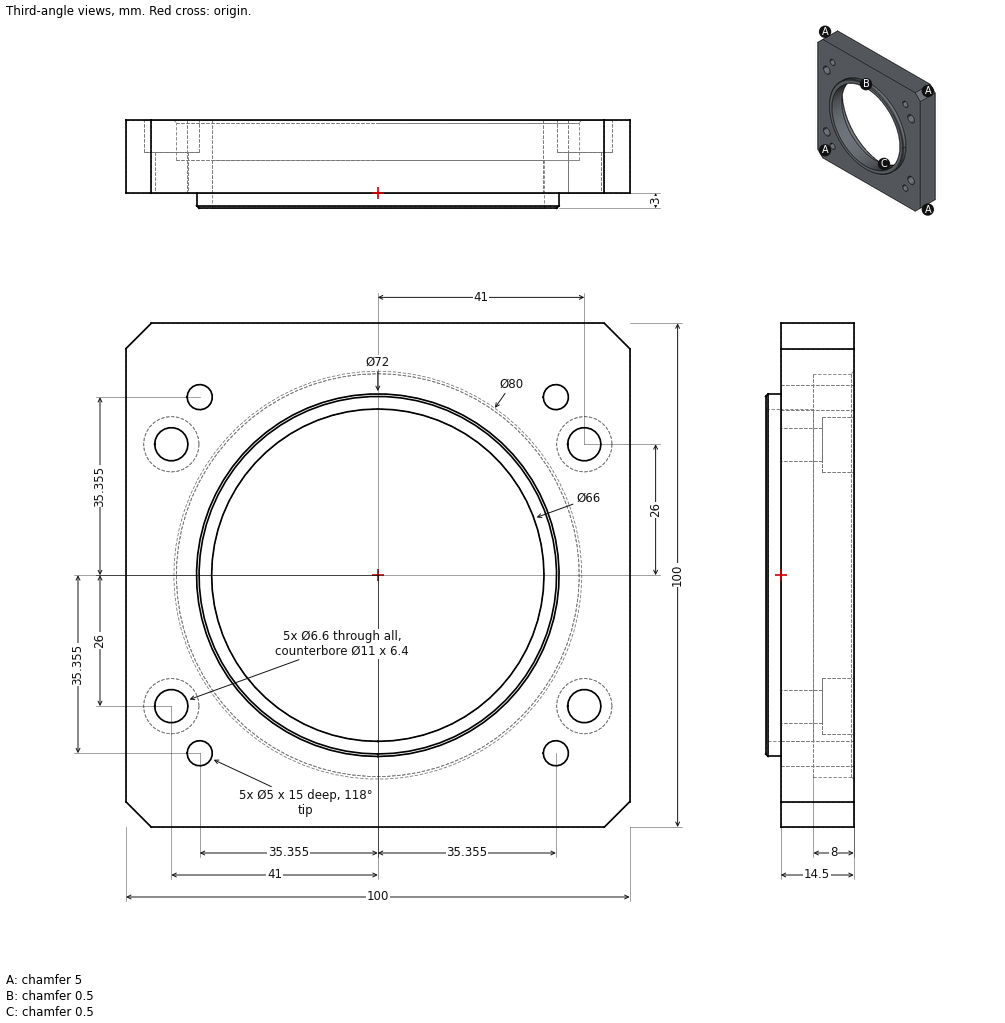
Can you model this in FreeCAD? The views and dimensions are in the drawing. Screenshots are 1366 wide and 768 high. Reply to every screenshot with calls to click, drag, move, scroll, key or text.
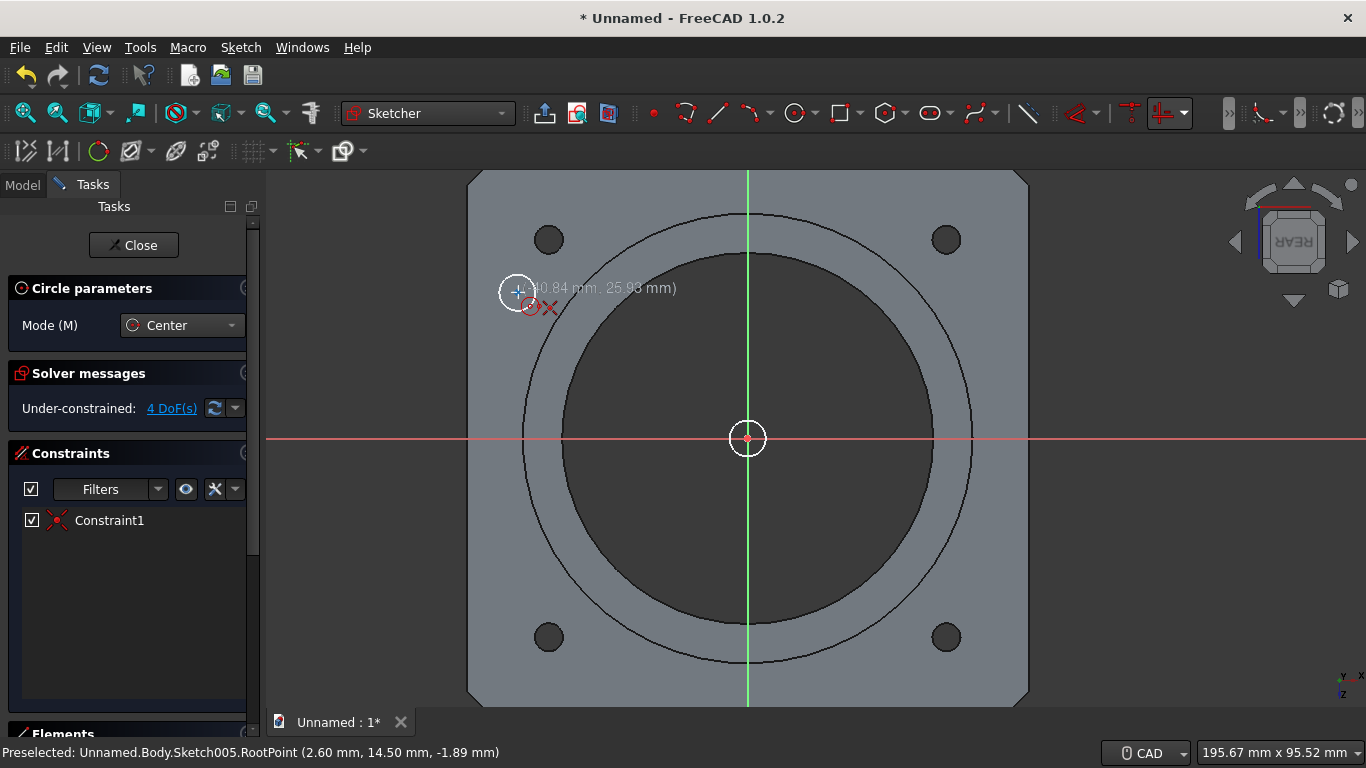
scroll(978, 585, up, 2)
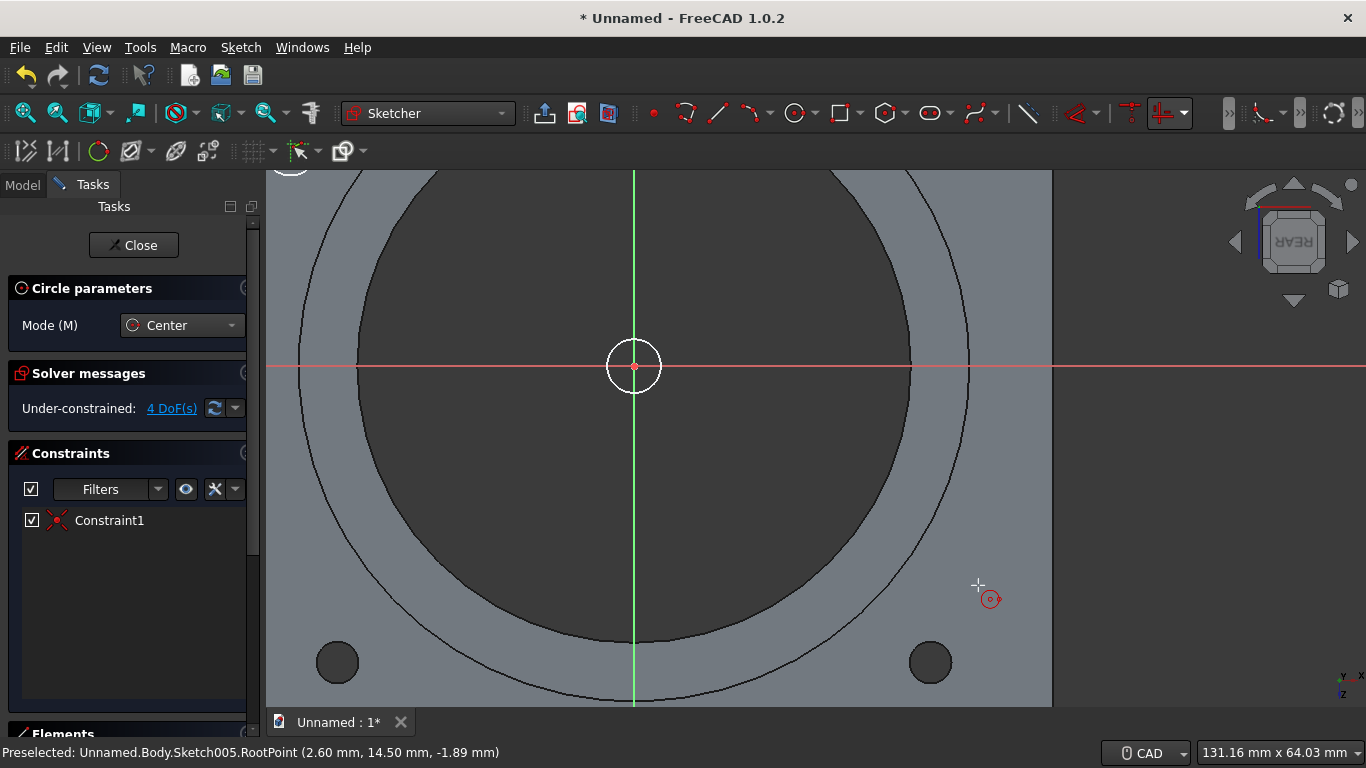
click(978, 584)
click(997, 565)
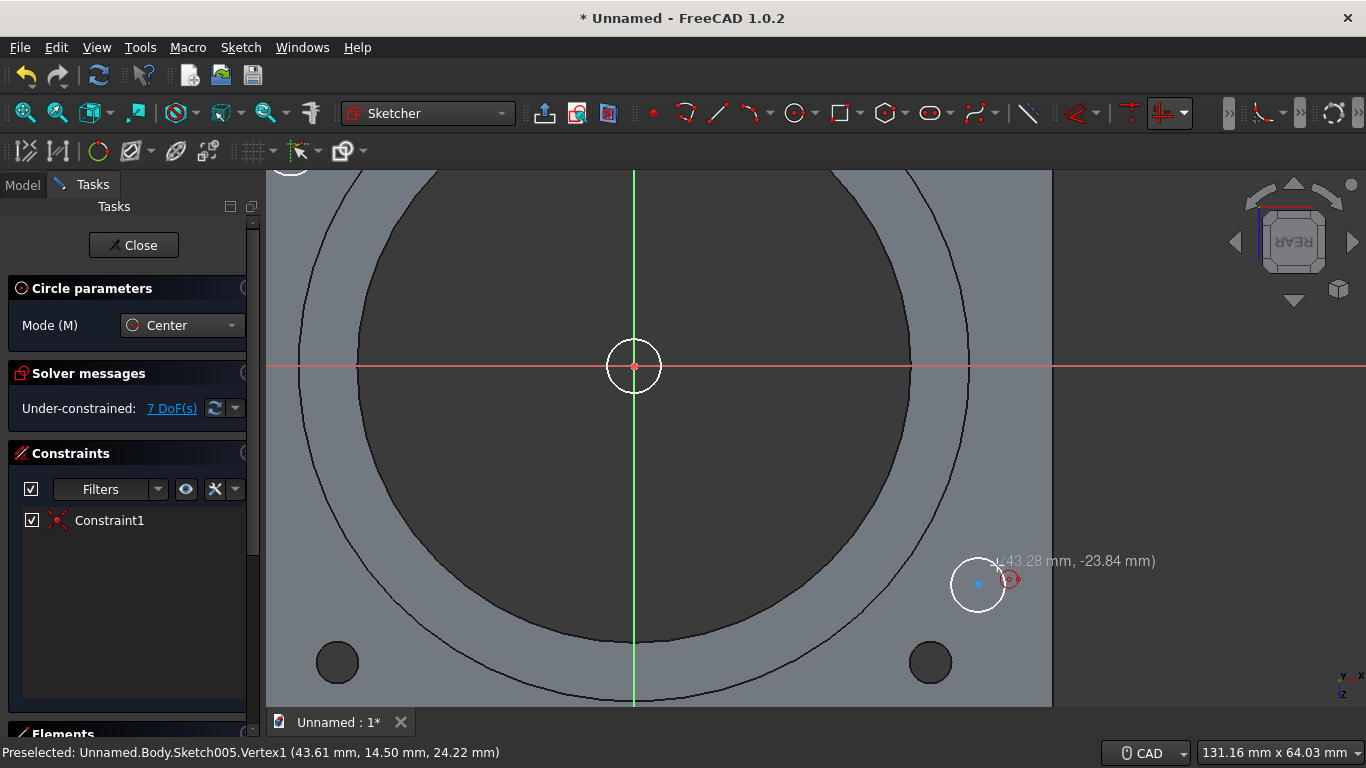
scroll(978, 586, down, 2)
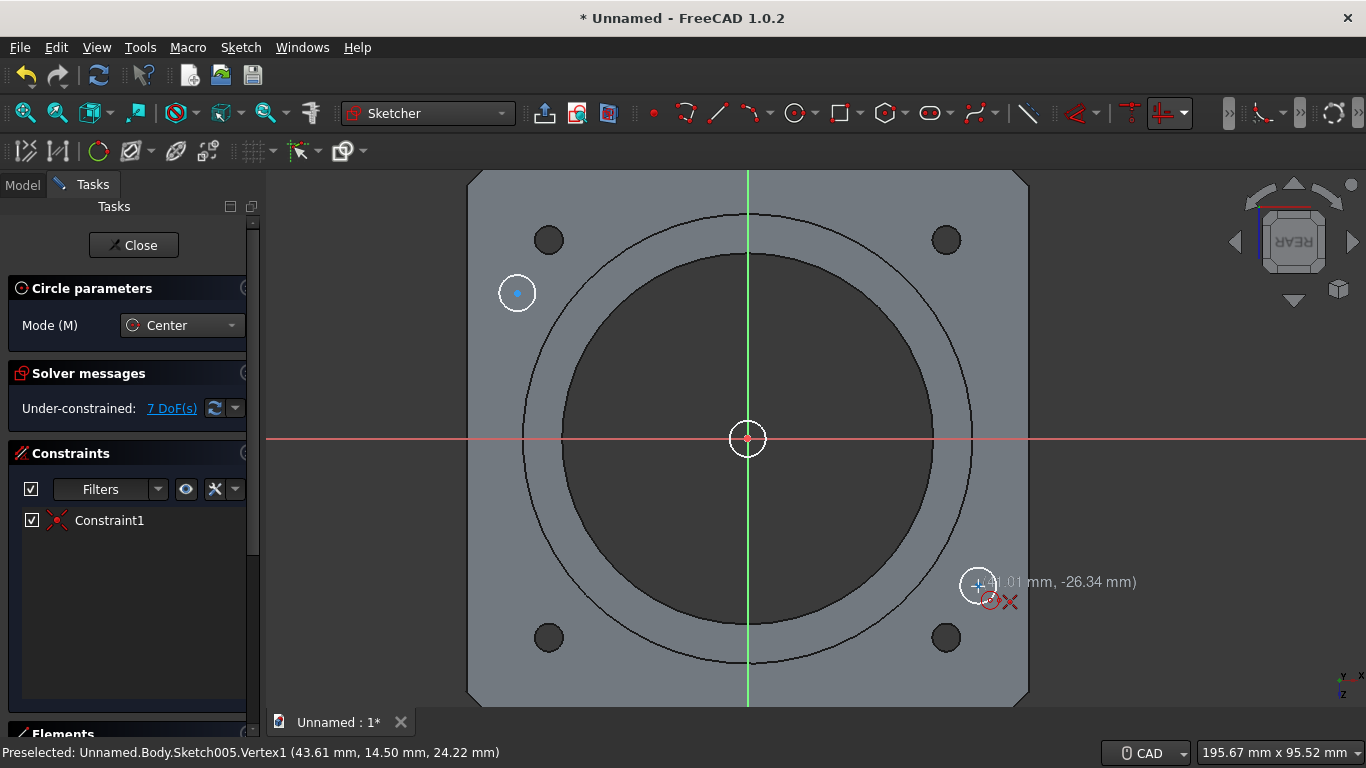
scroll(978, 293, up, 2)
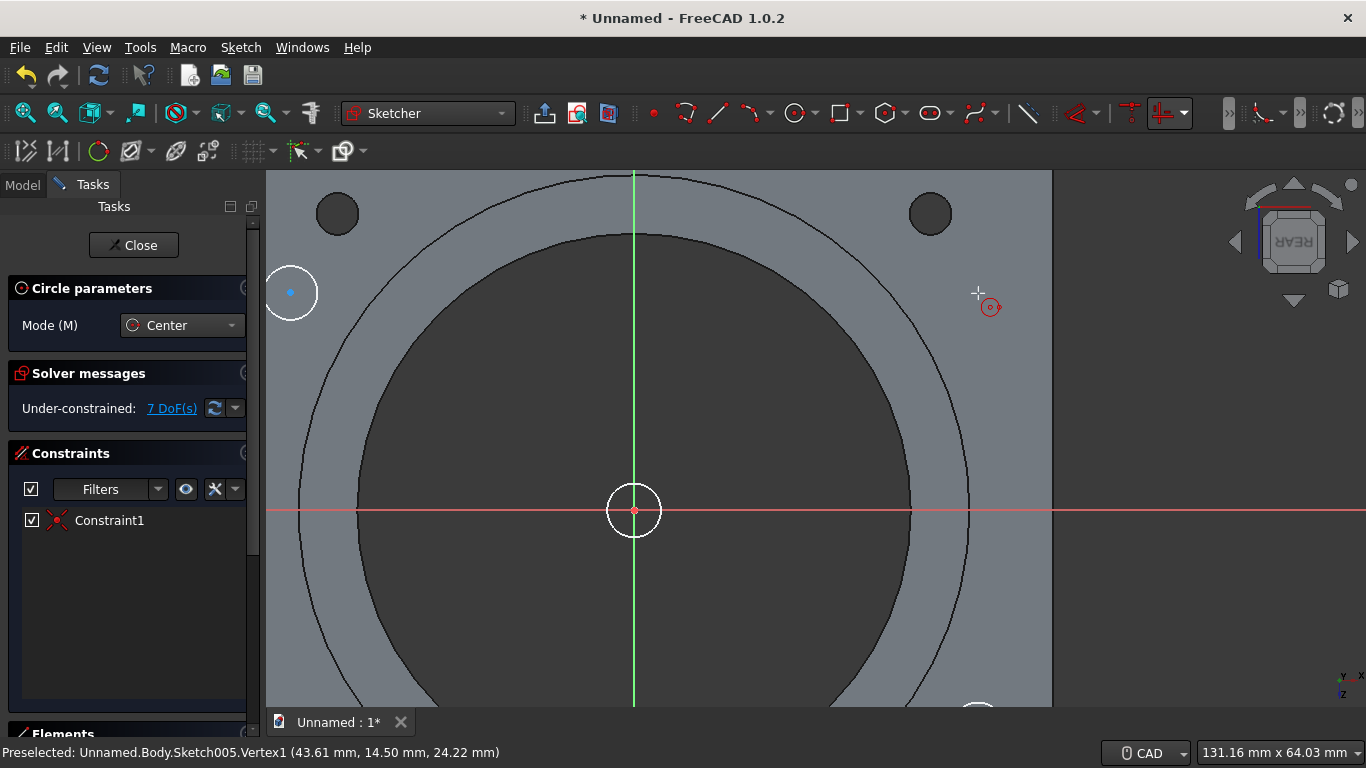
click(978, 292)
click(997, 273)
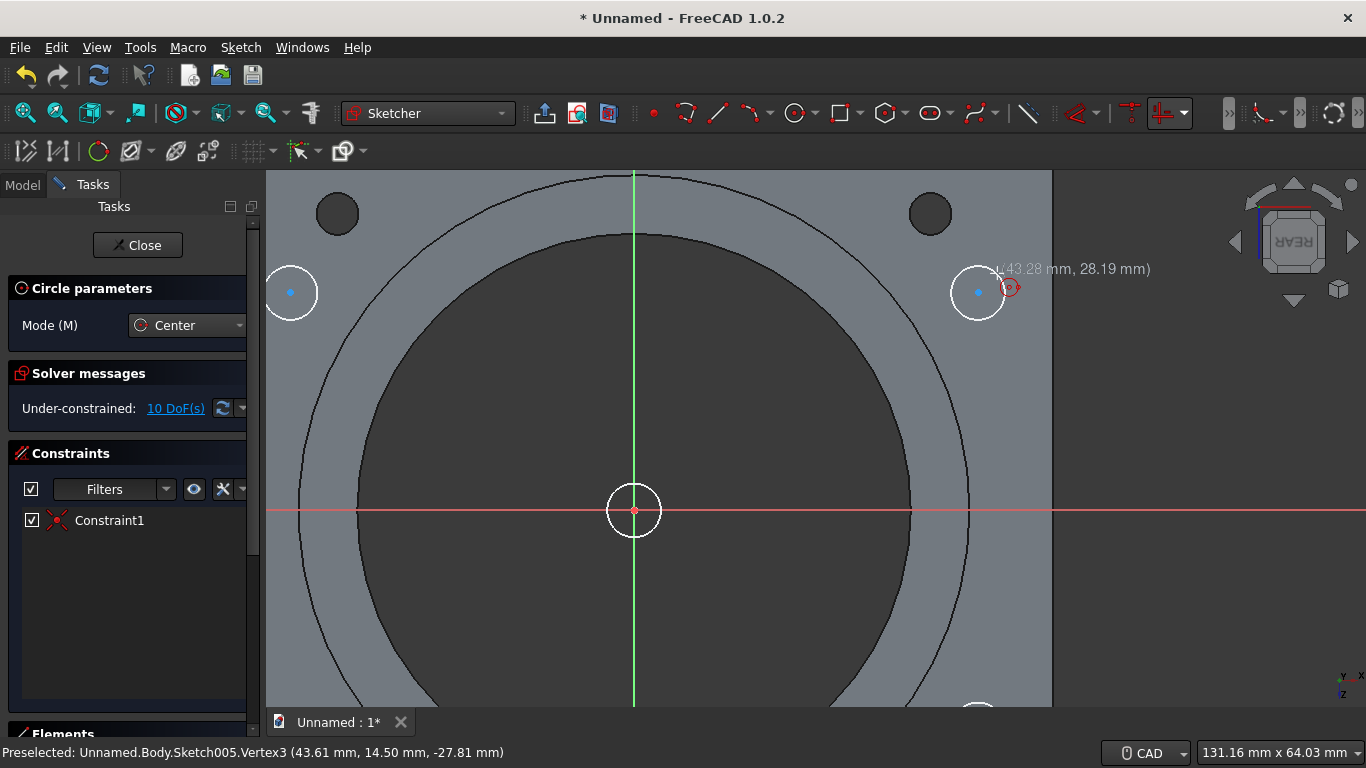
scroll(978, 292, down, 2)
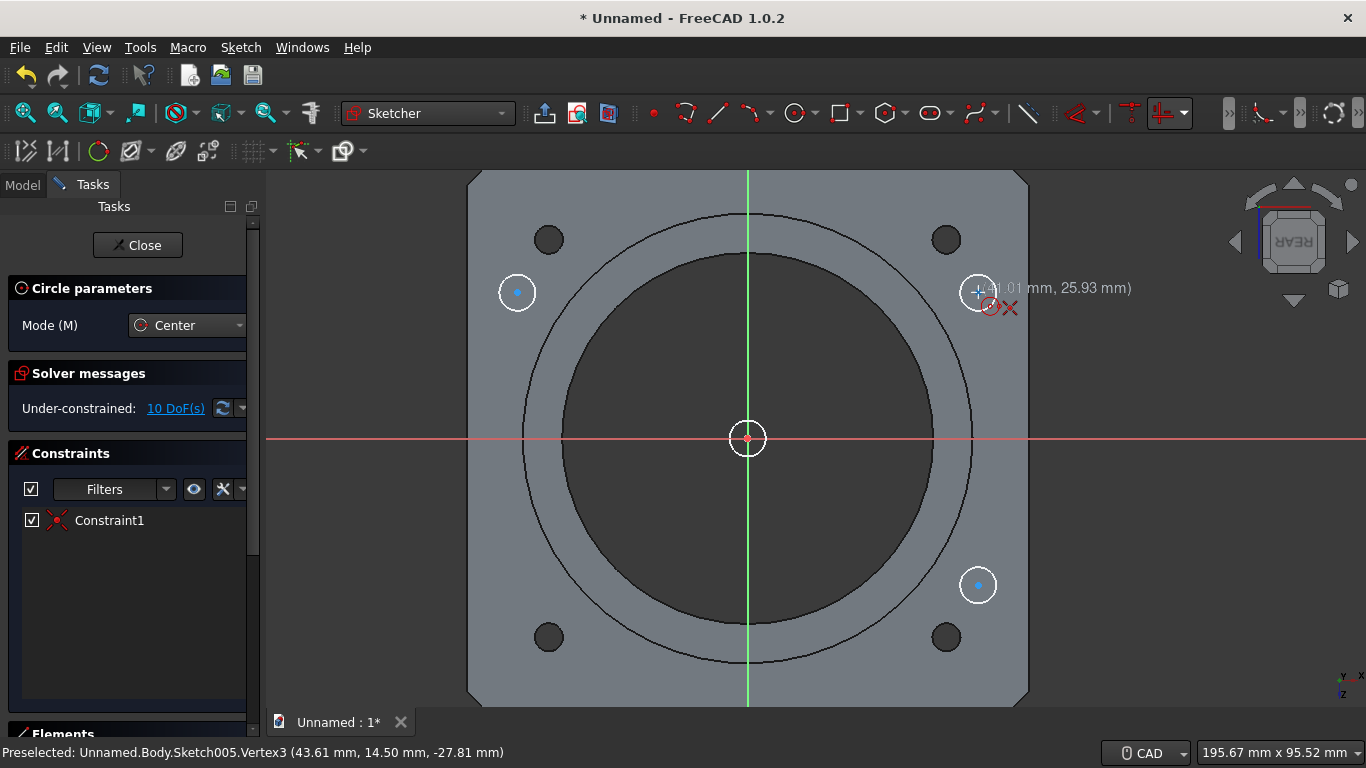
scroll(517, 585, up, 2)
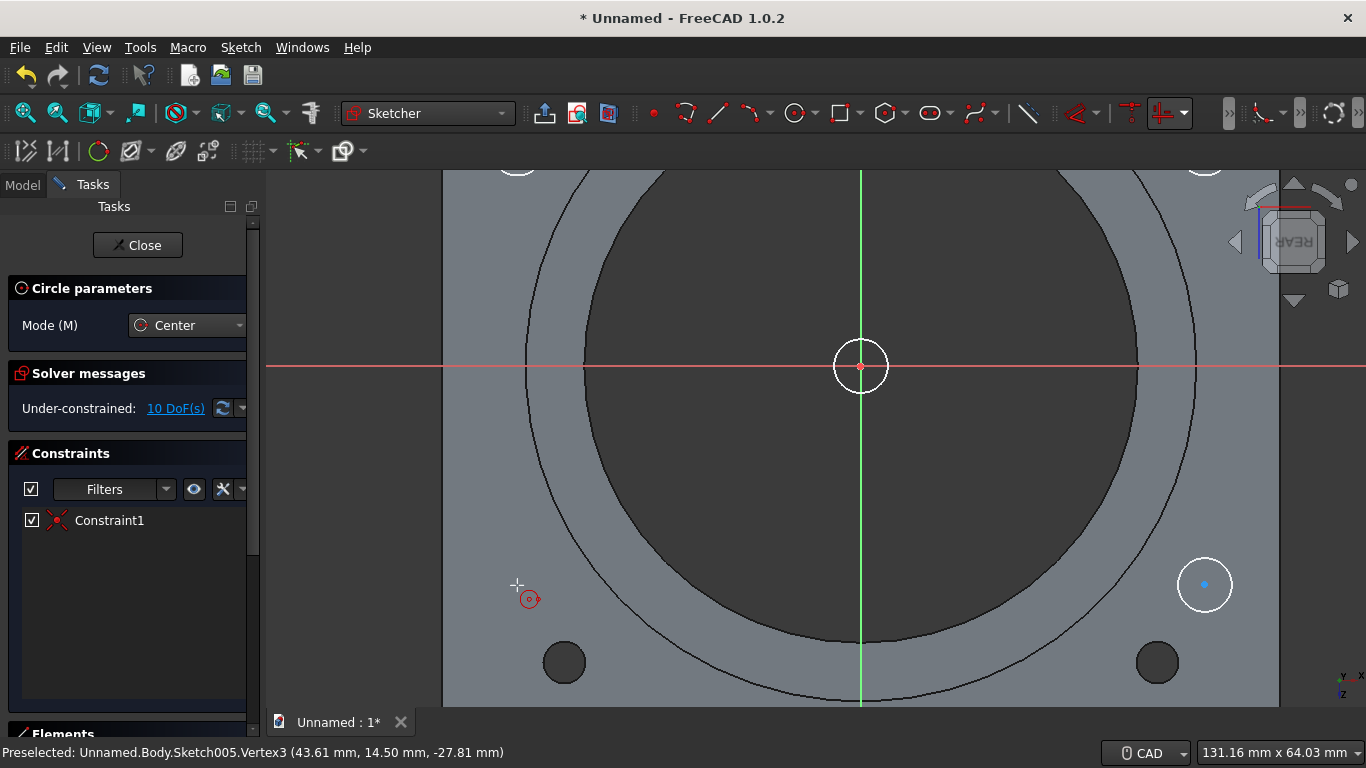
click(517, 584)
click(537, 565)
key(Escape)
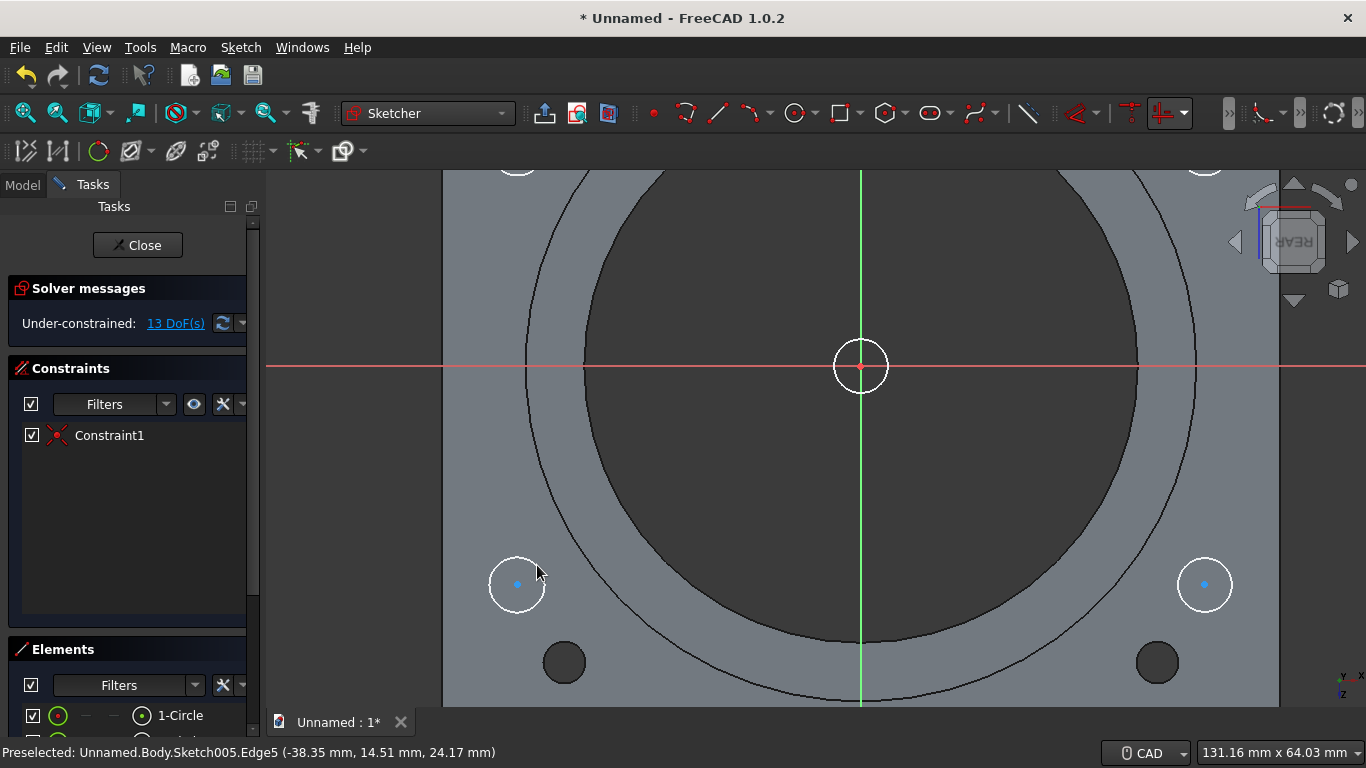
scroll(517, 586, down, 2)